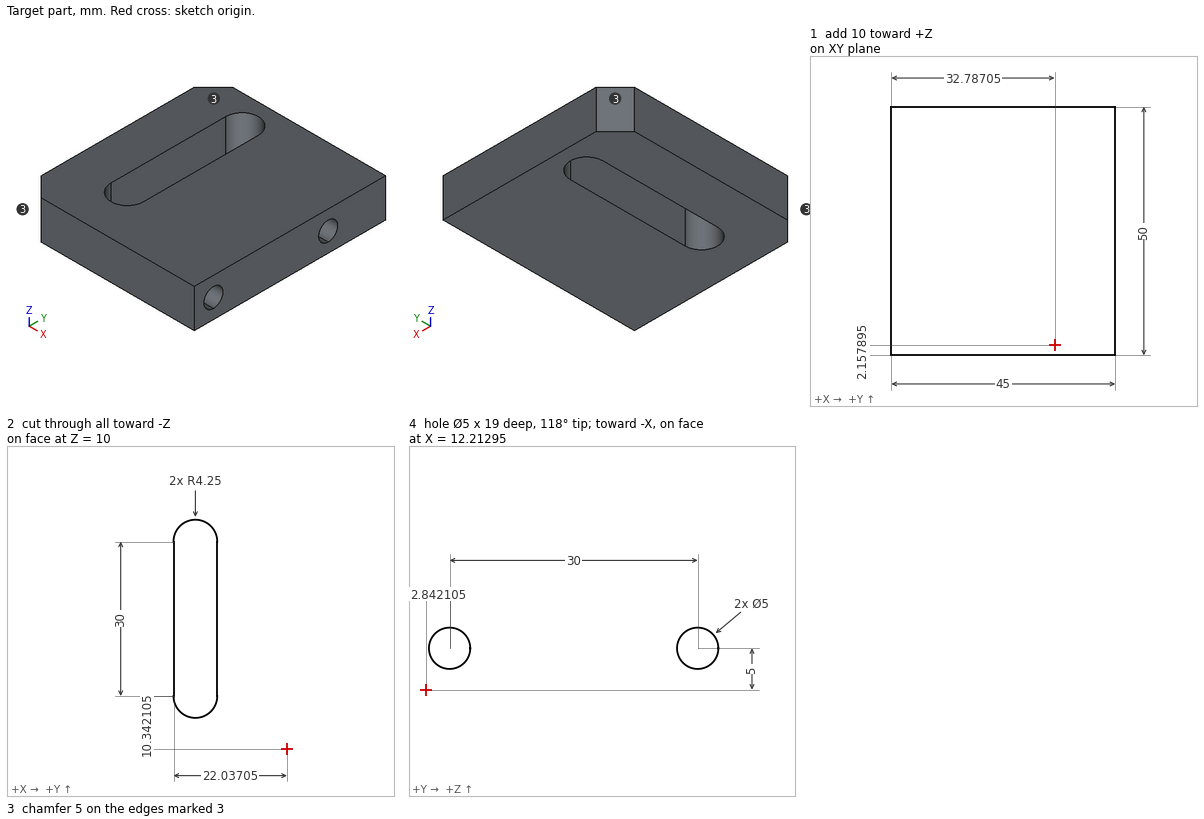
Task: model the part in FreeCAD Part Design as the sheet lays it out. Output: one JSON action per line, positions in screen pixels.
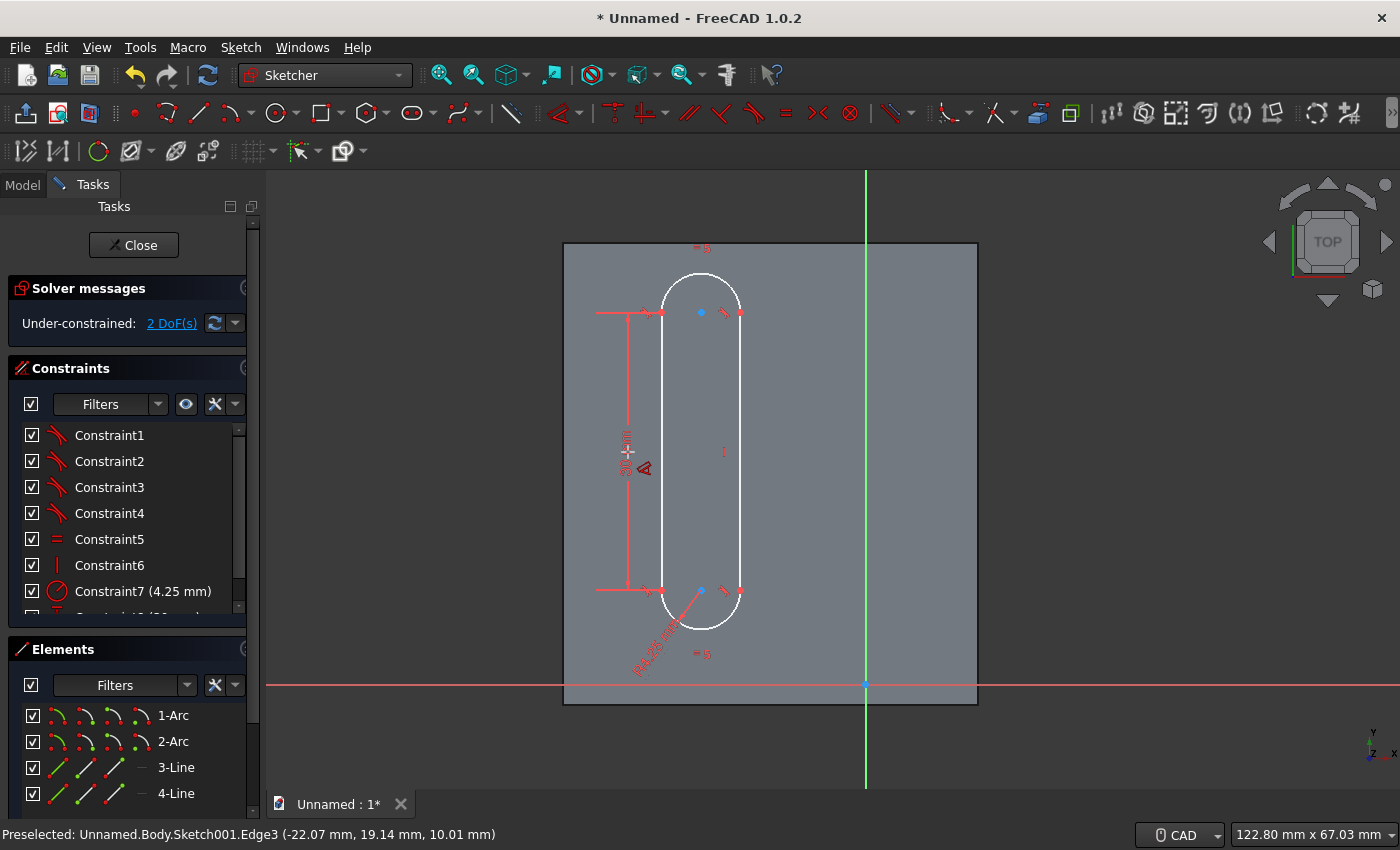
{"action": "left_click", "coordinate": [662, 590]}
{"action": "left_click", "coordinate": [764, 719]}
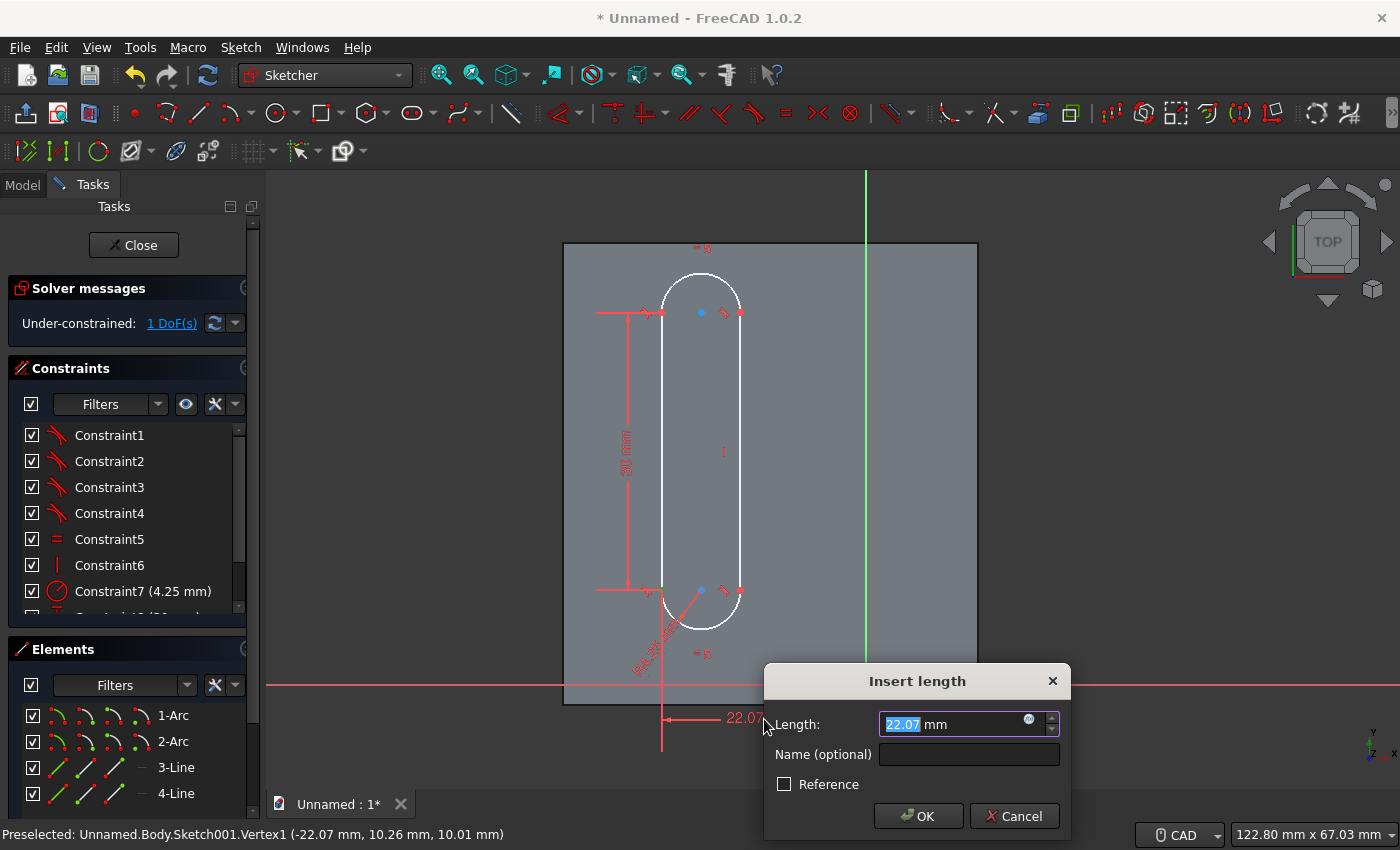
{"action": "type", "text": "22.03705"}
{"action": "key", "text": "Return"}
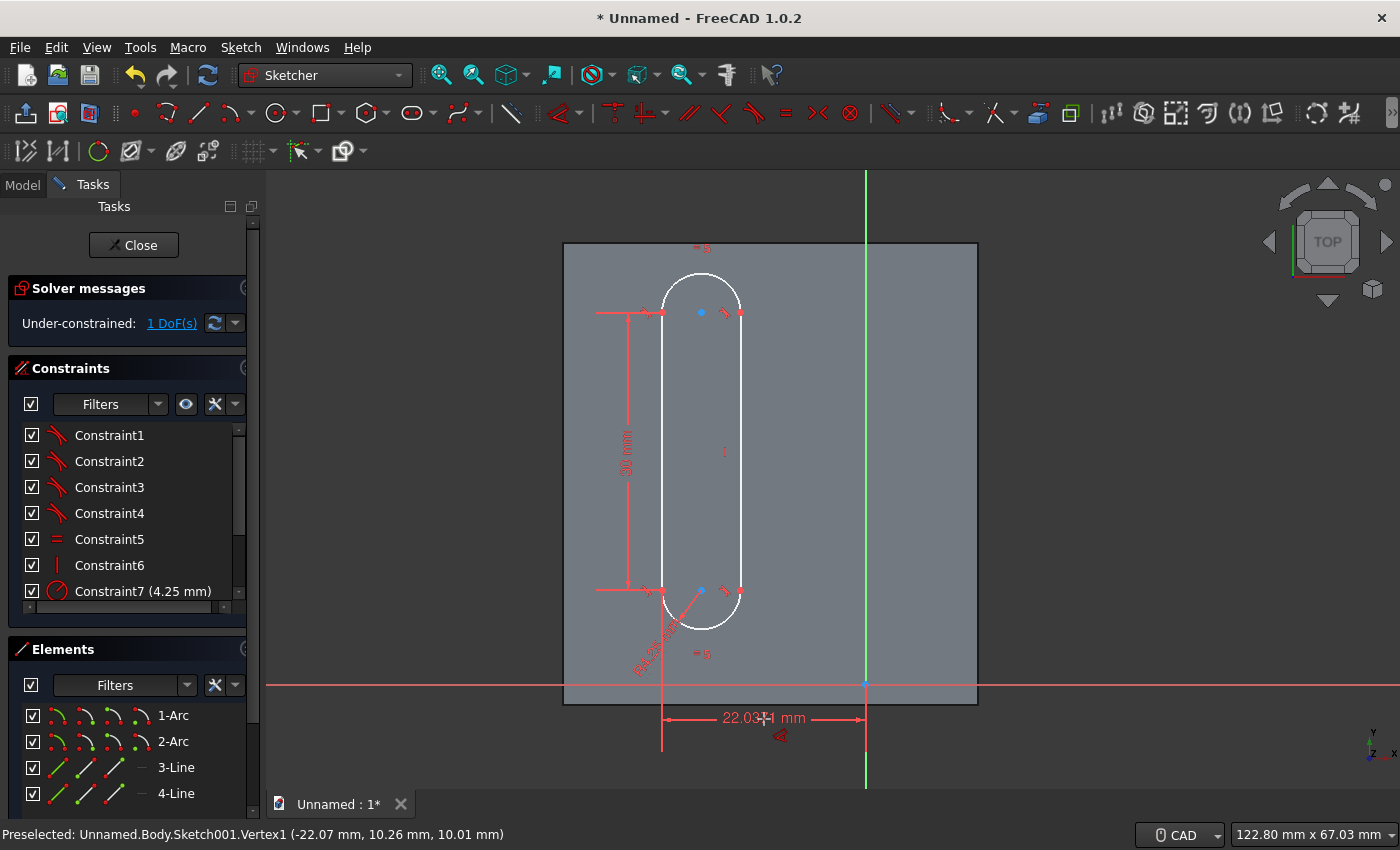
{"action": "left_click", "coordinate": [662, 590]}
{"action": "left_click", "coordinate": [628, 616]}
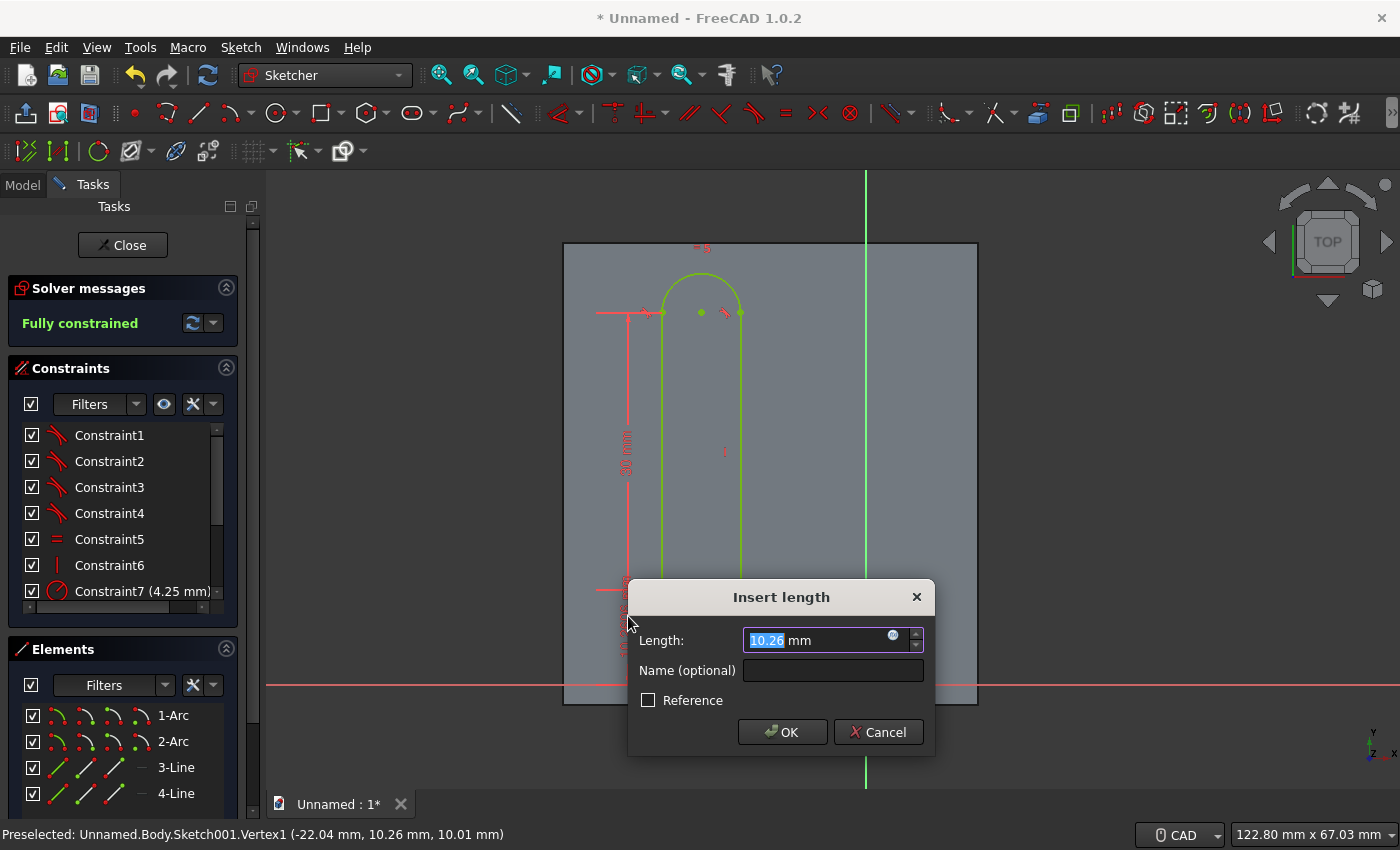
{"action": "type", "text": "10.342105"}
{"action": "key", "text": "Return"}
{"action": "key", "text": "Escape"}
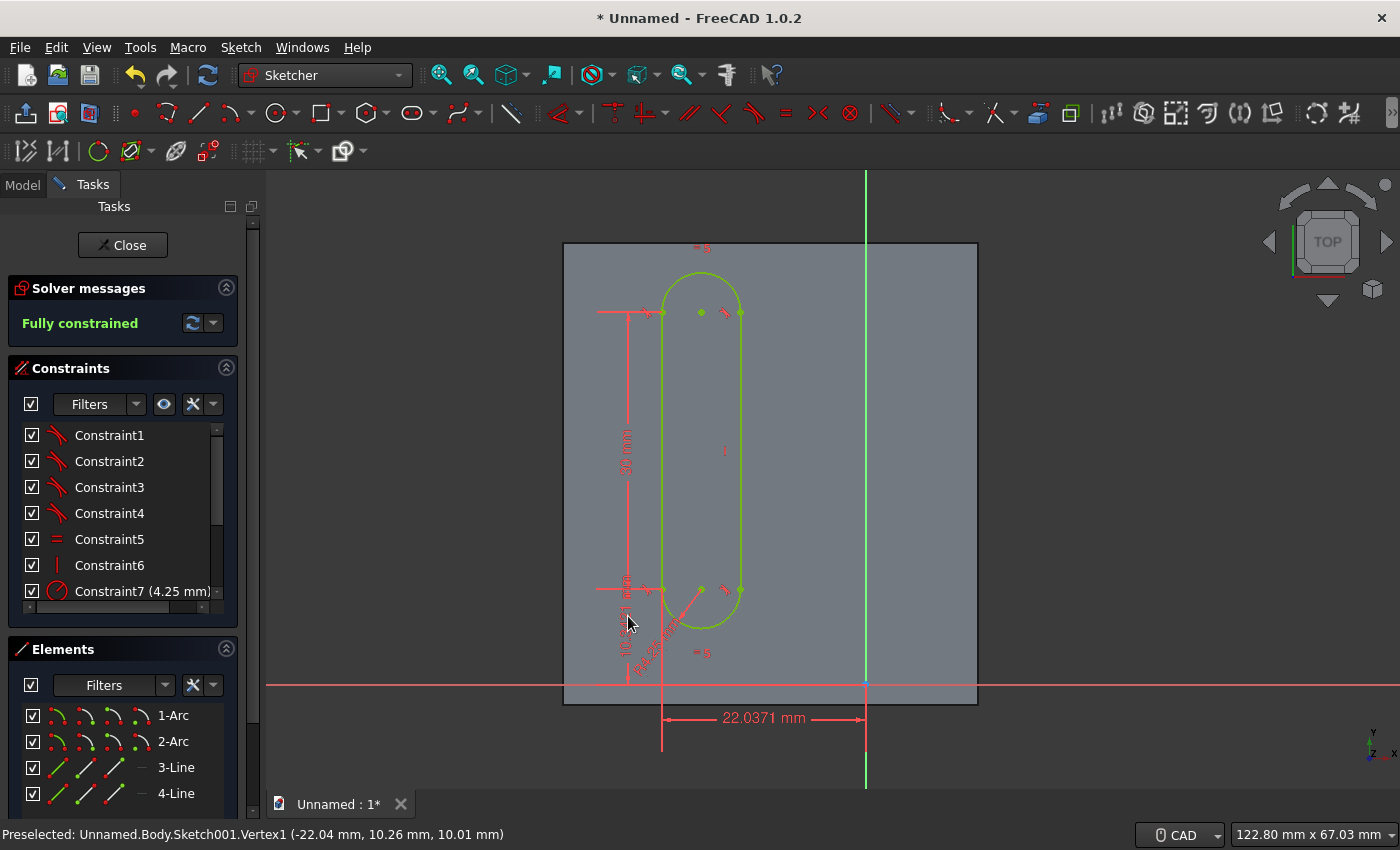
{"action": "left_click", "coordinate": [123, 245]}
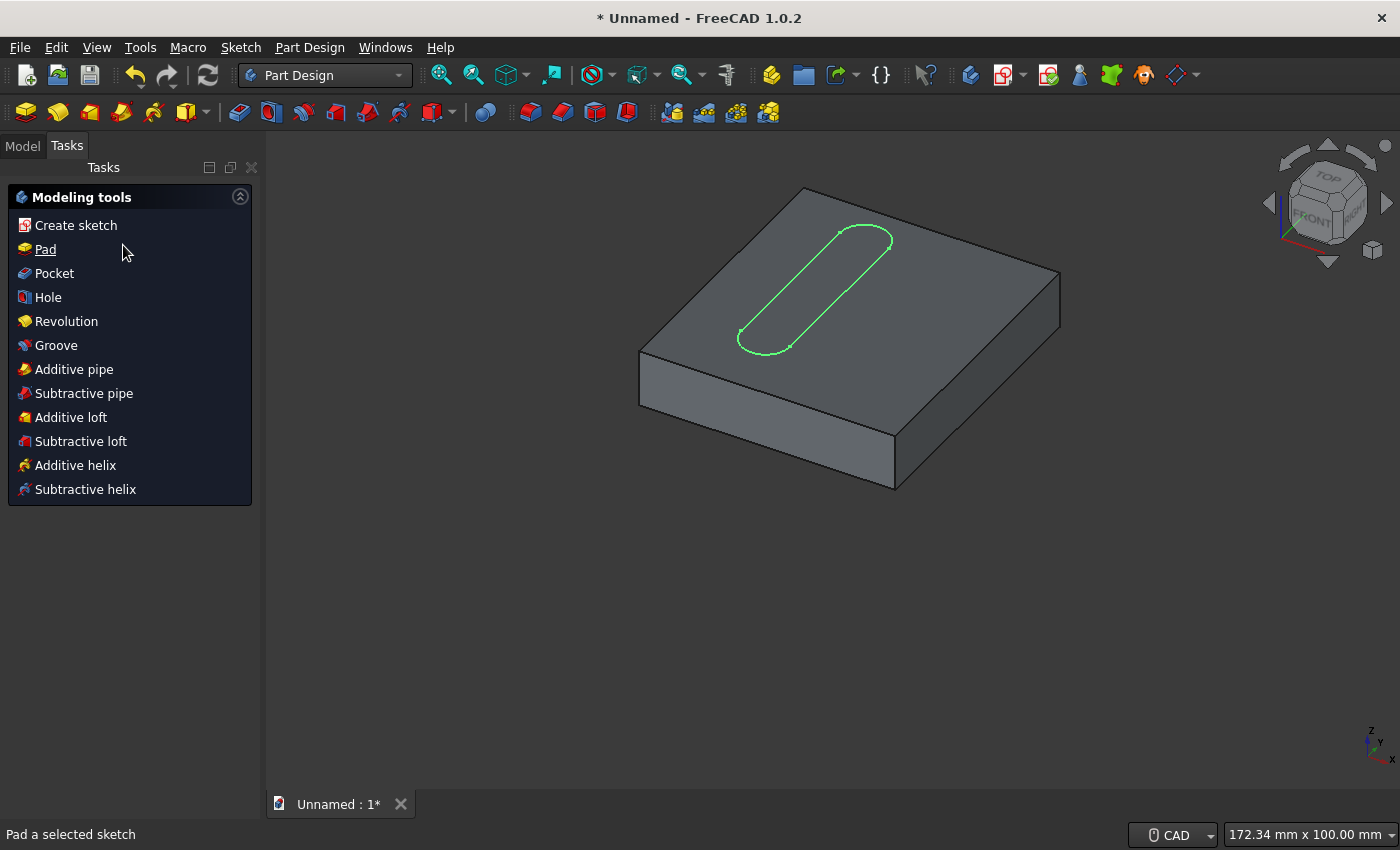
{"action": "left_click", "coordinate": [240, 112]}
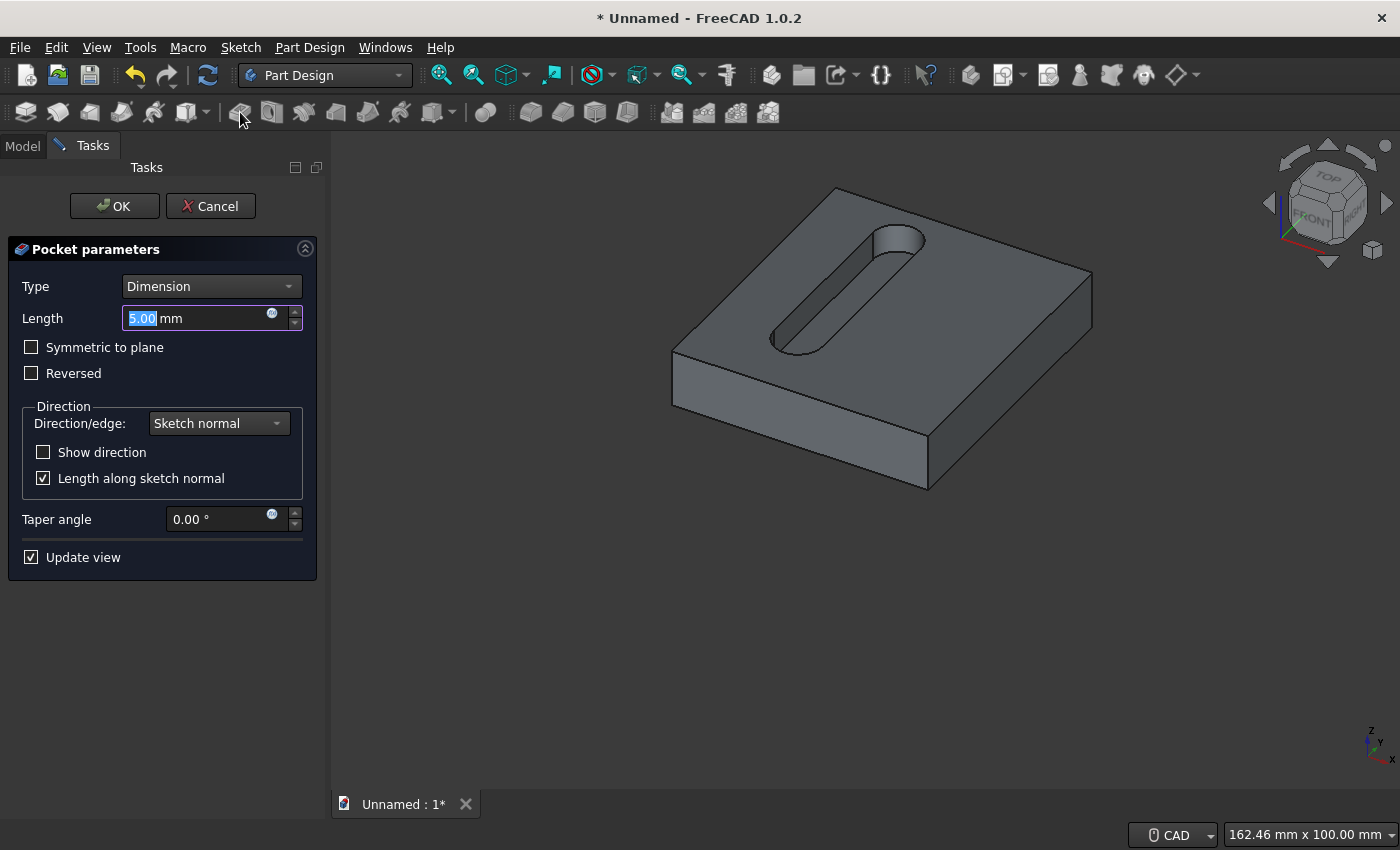
{"action": "left_click", "coordinate": [212, 286]}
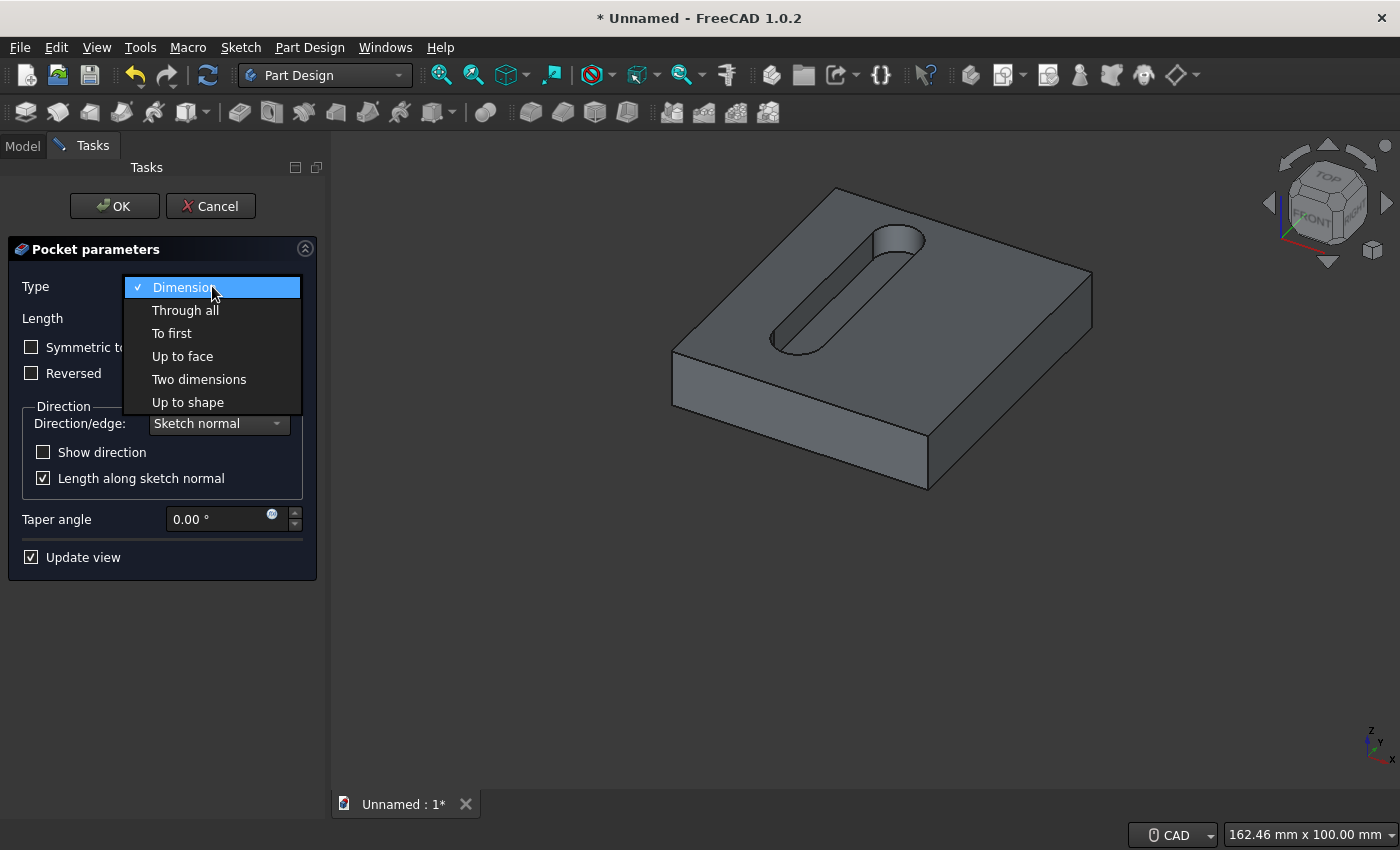
{"action": "left_click", "coordinate": [212, 310]}